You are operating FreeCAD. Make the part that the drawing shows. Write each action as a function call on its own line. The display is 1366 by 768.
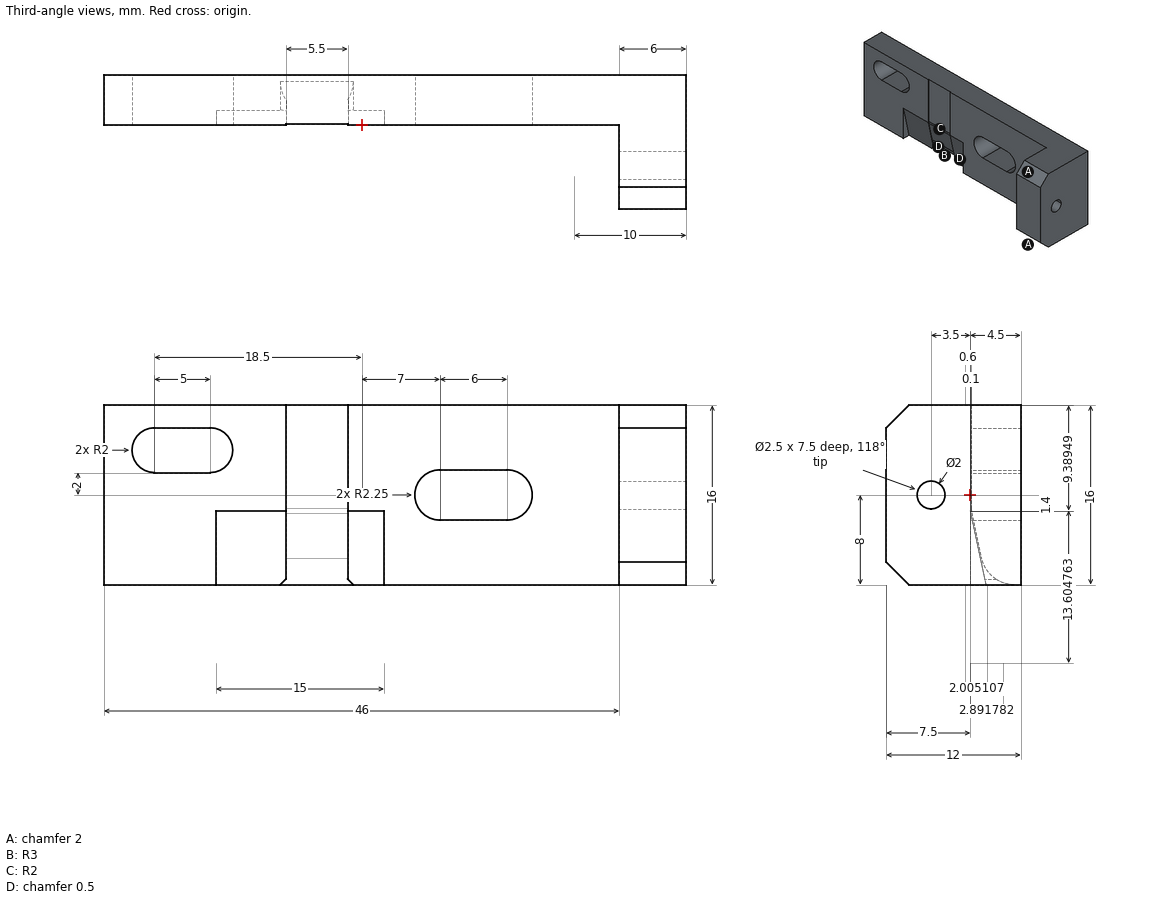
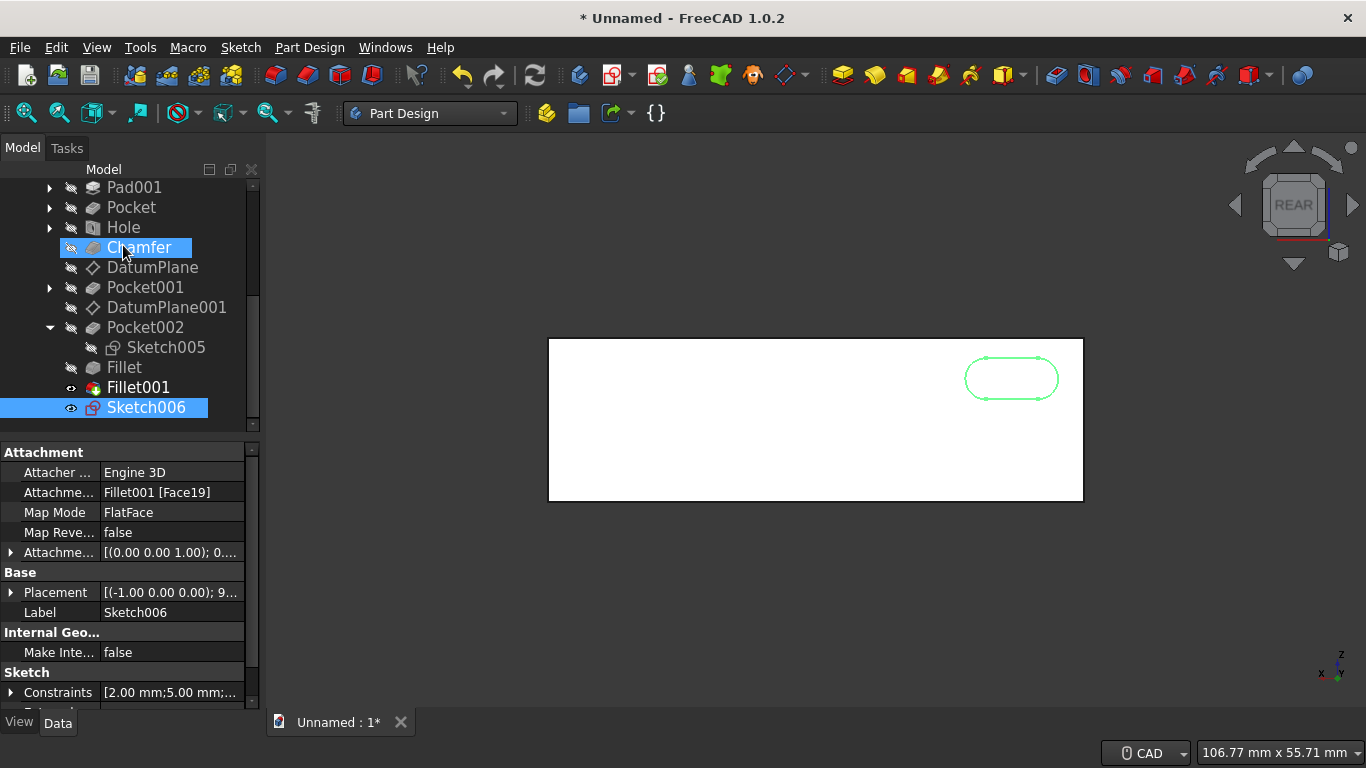
click(1058, 76)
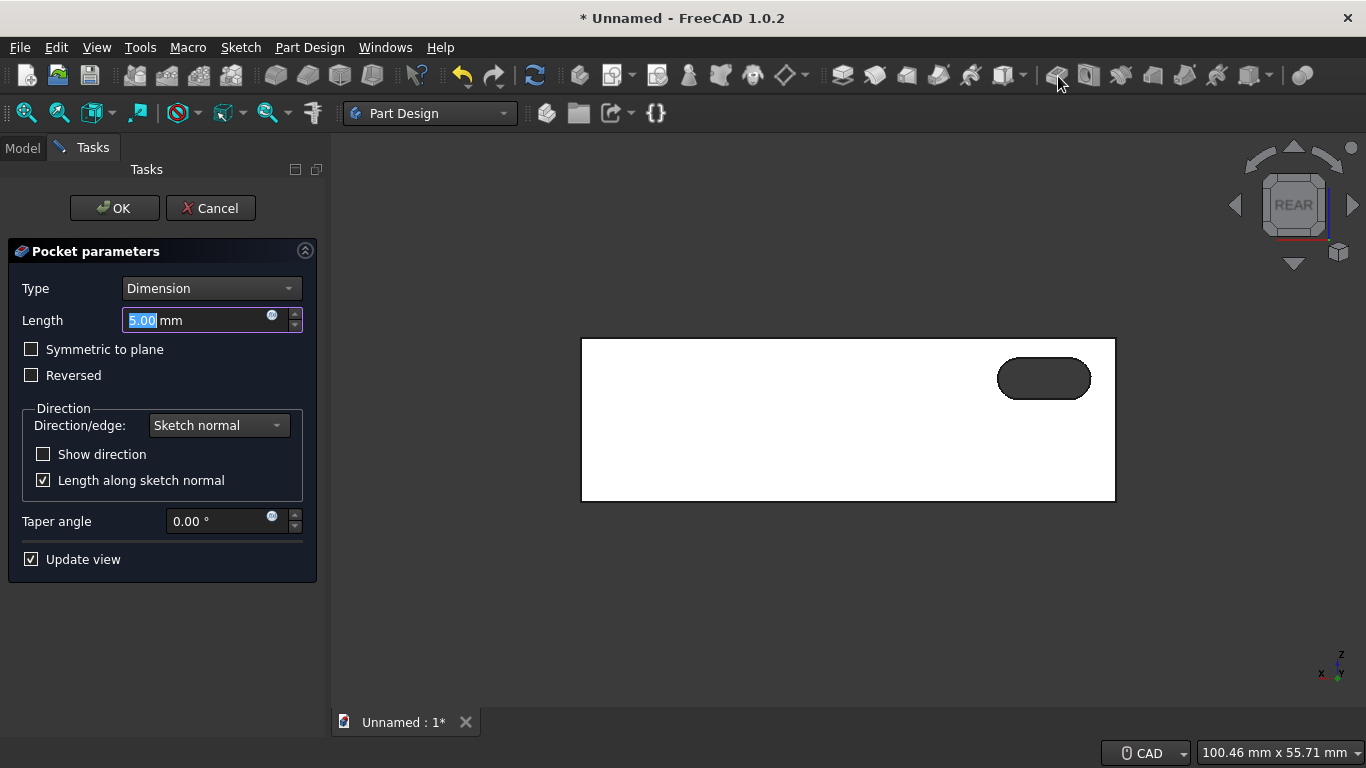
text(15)
key(Tab)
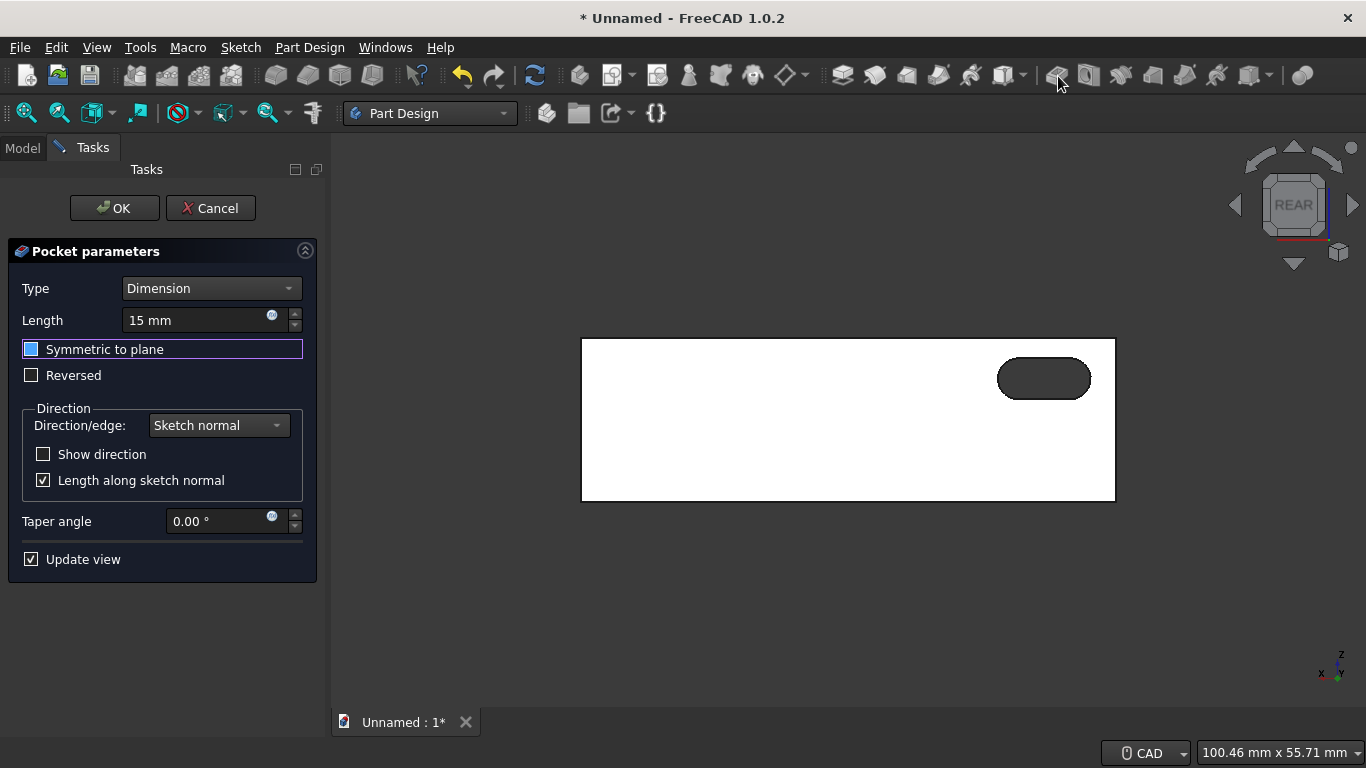
click(115, 208)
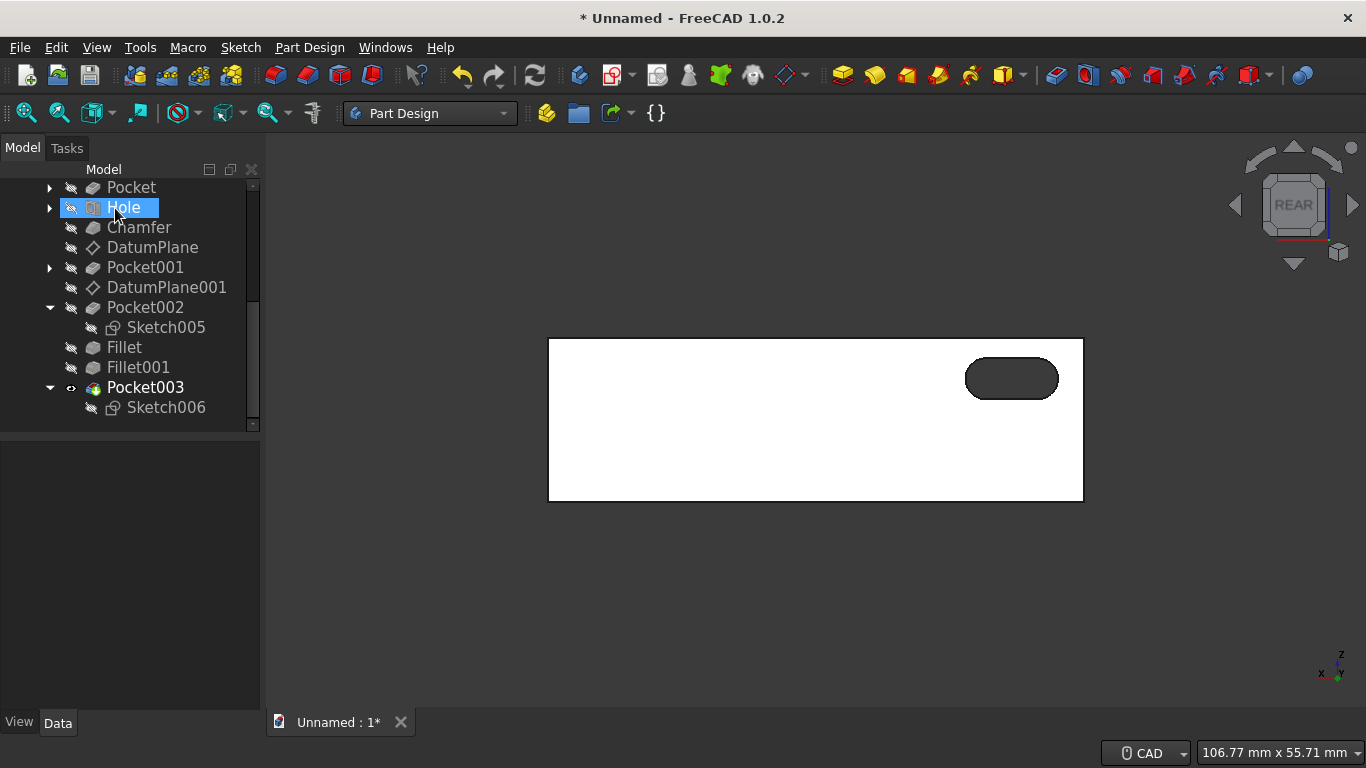
click(663, 419)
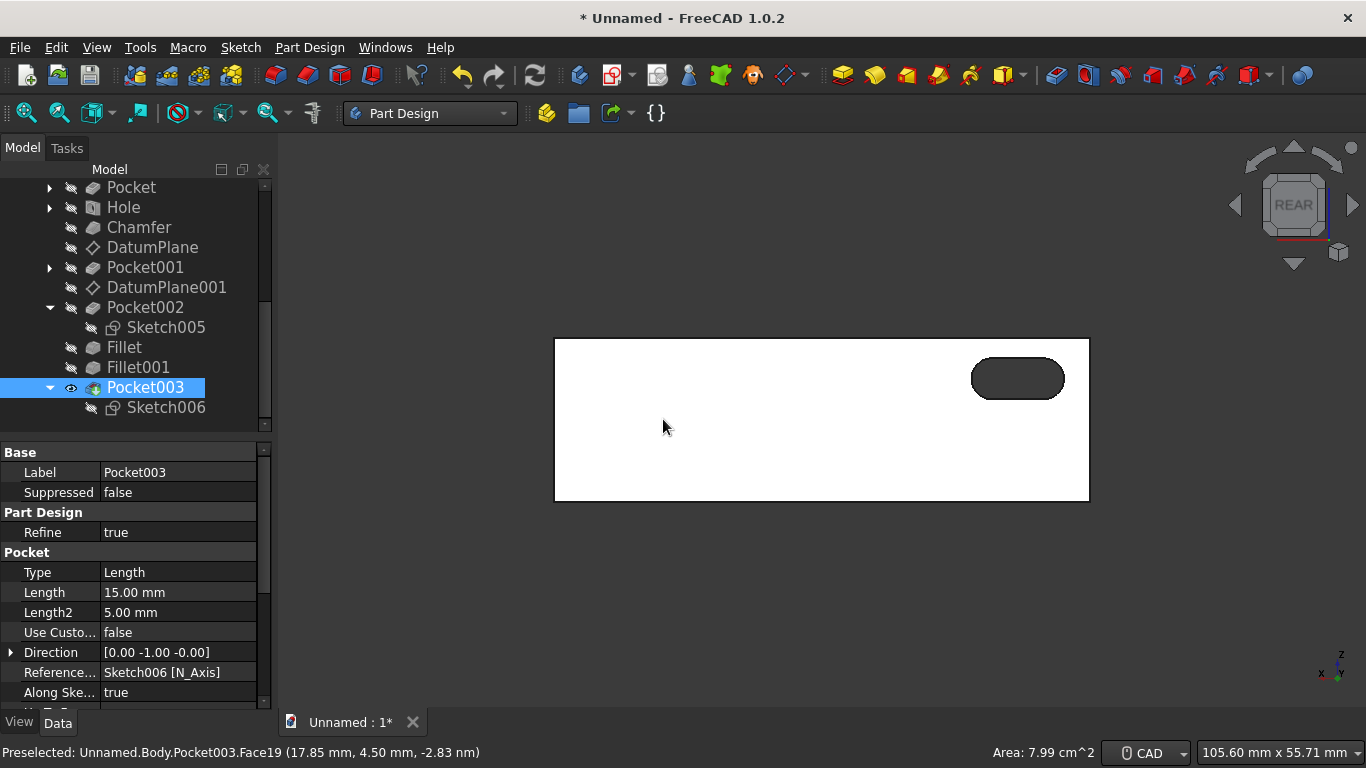
click(612, 76)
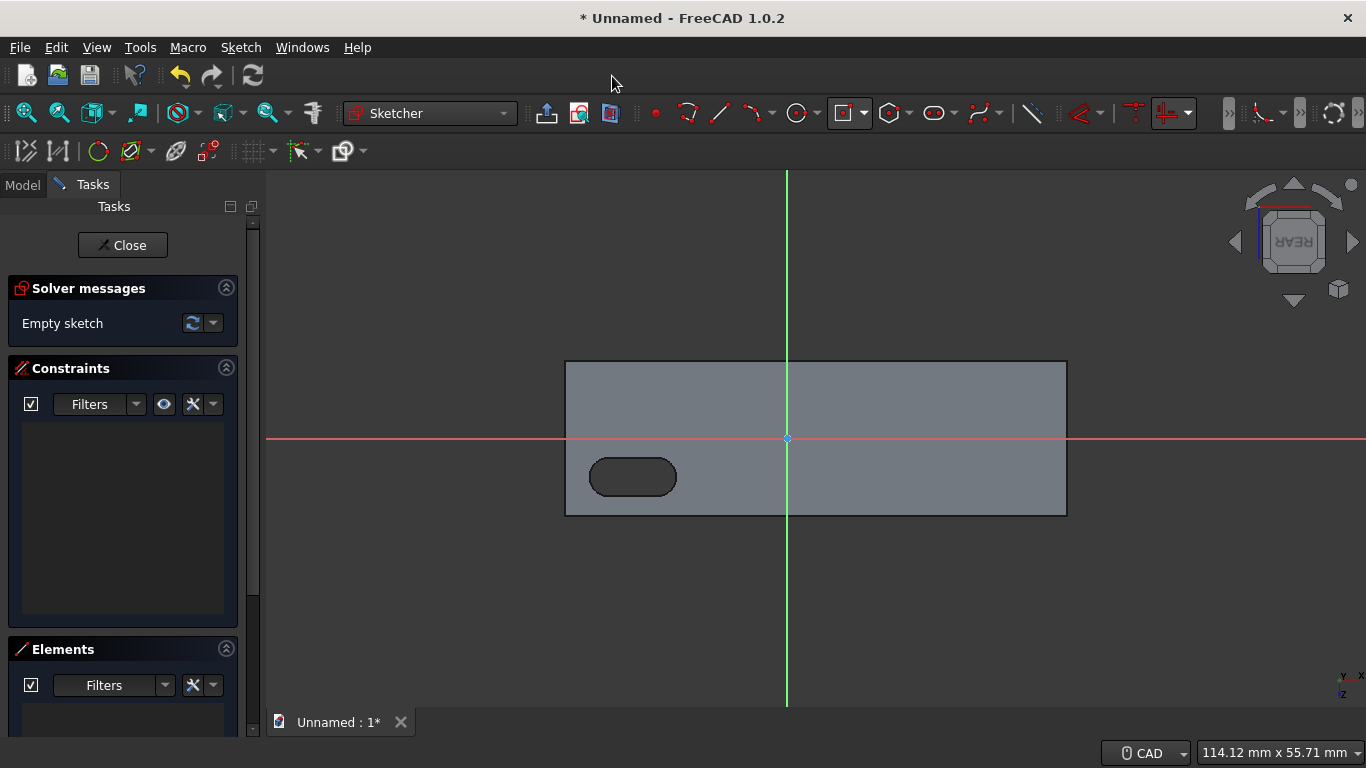
scroll(898, 438, up, 7)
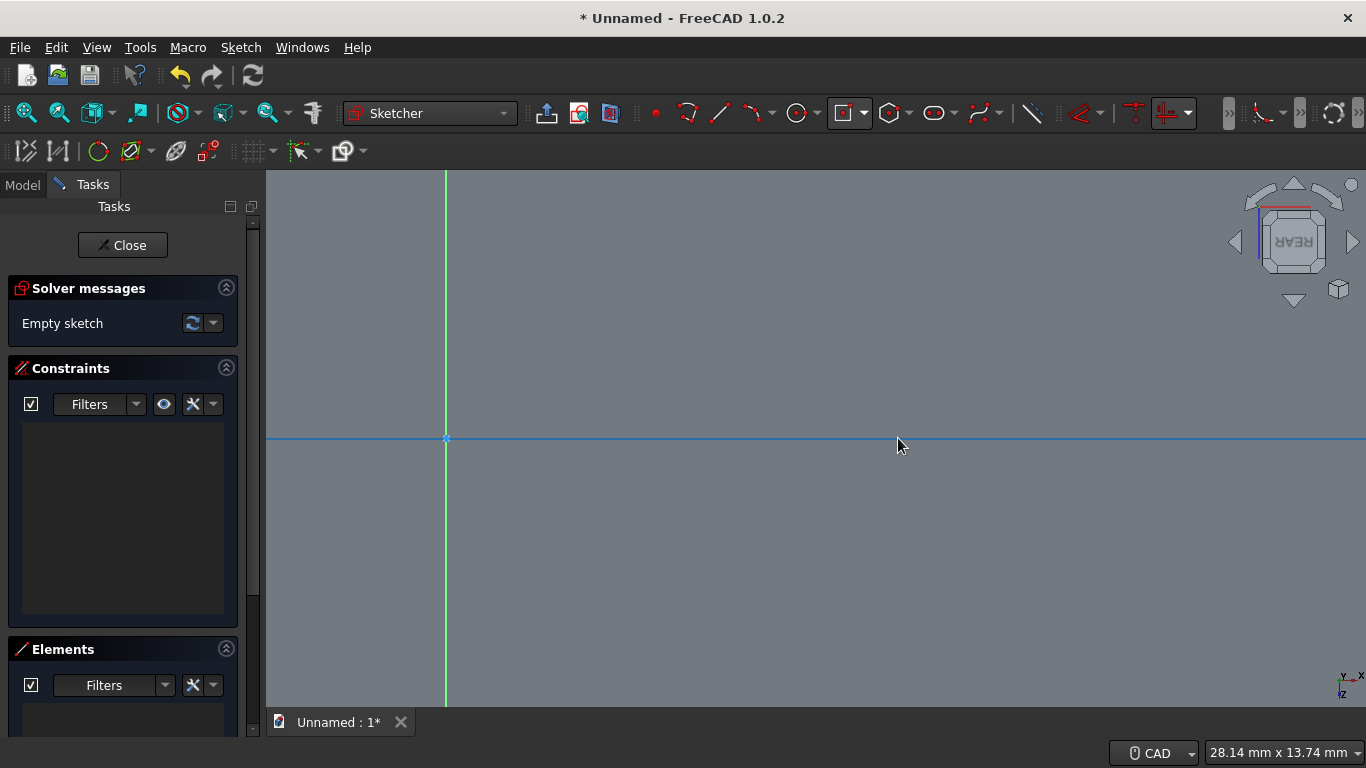
key(g)
key(s)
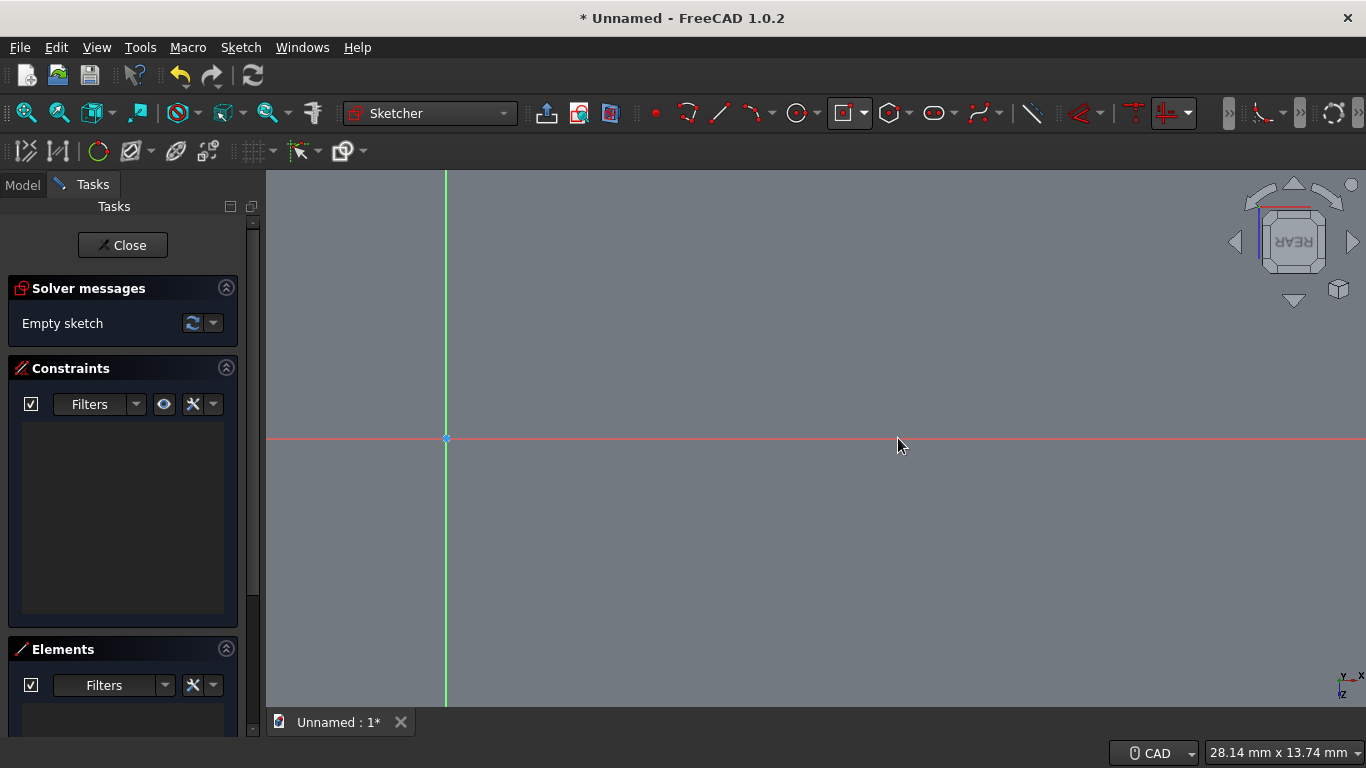
click(720, 438)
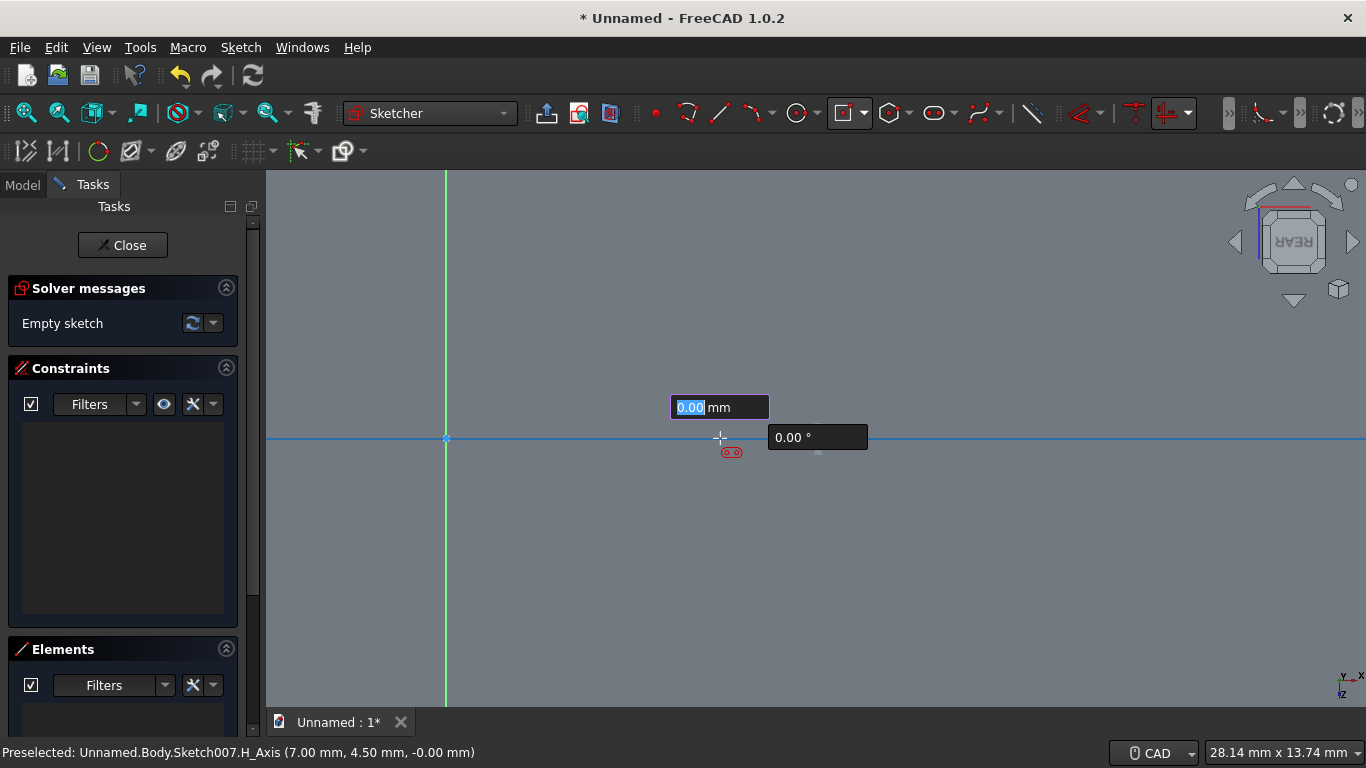
click(955, 429)